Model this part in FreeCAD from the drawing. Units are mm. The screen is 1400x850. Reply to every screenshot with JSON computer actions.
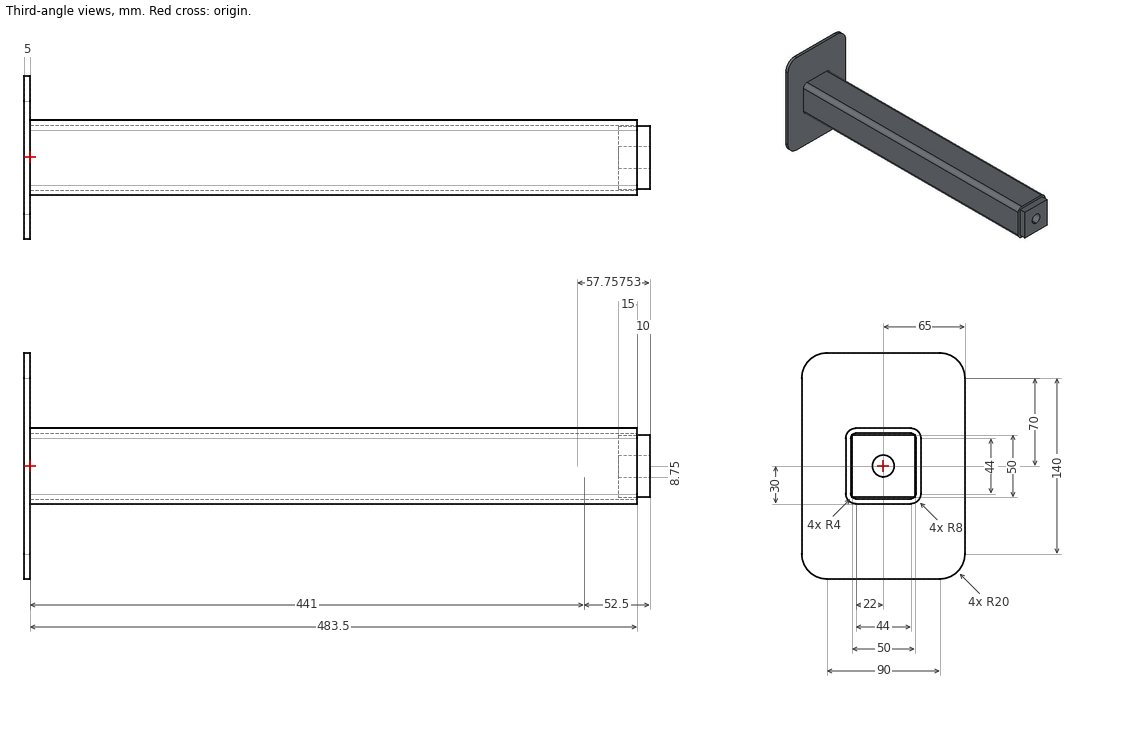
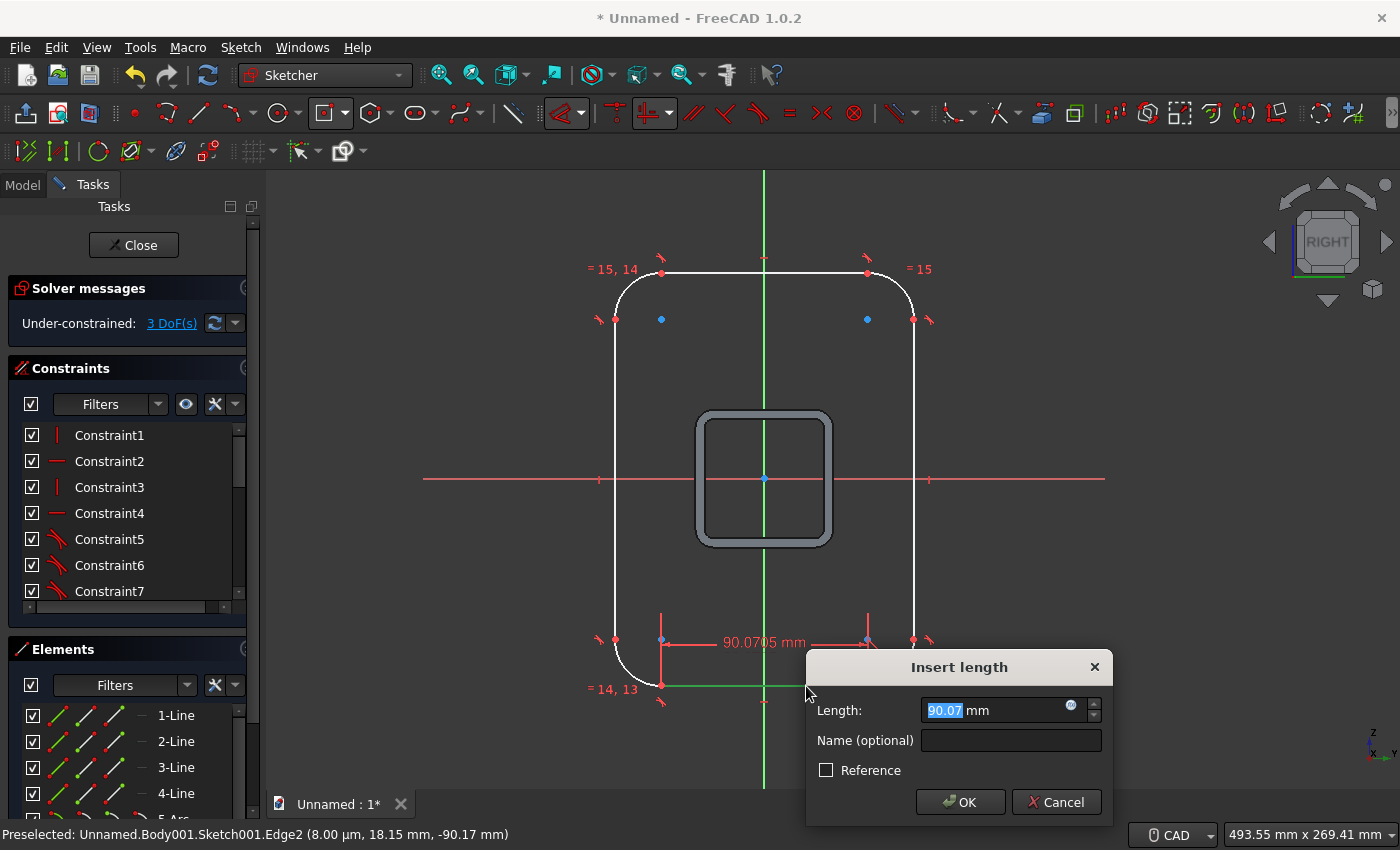
{"action": "type", "text": "90"}
{"action": "key", "text": "Return"}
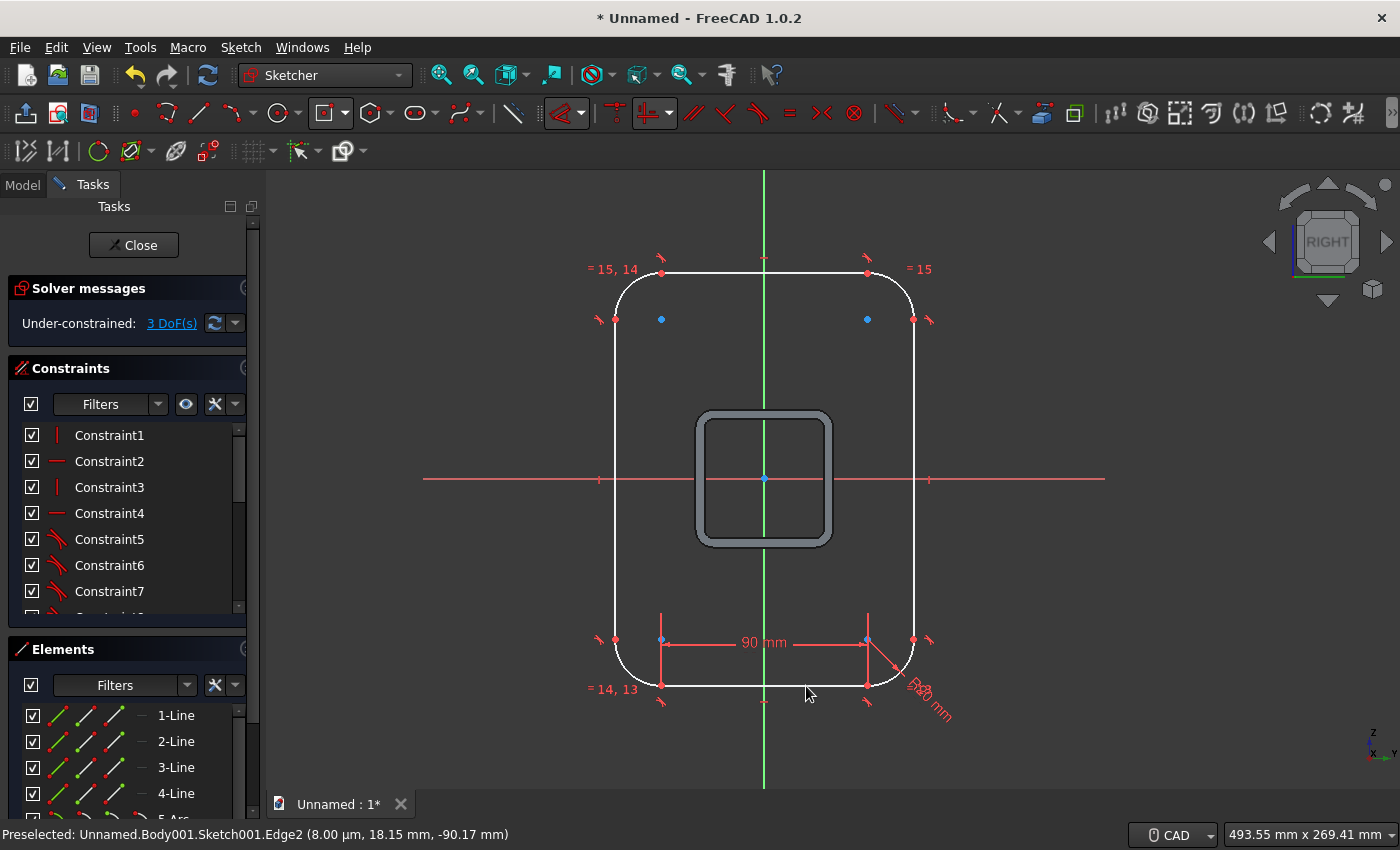
{"action": "left_click", "coordinate": [914, 415]}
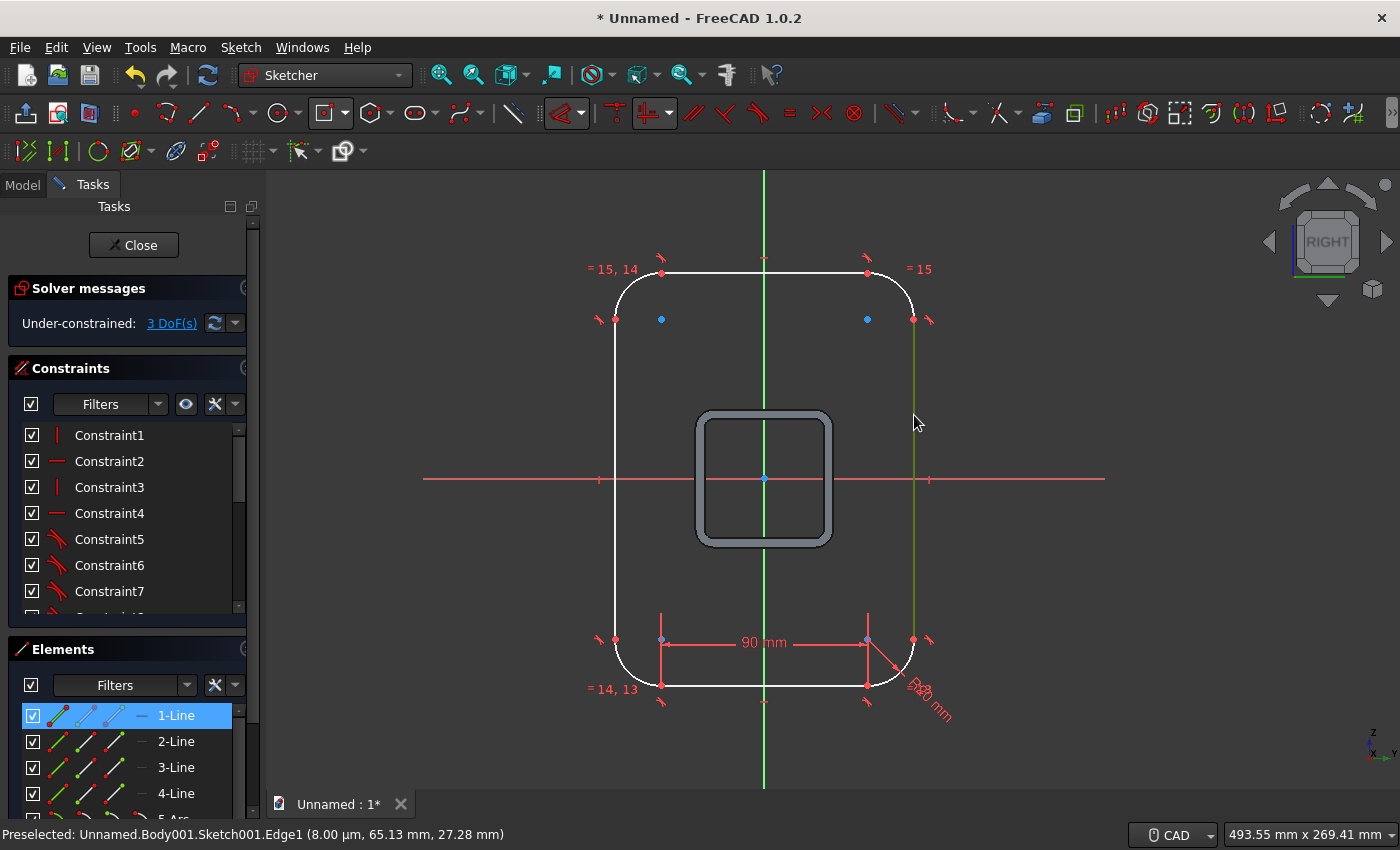
{"action": "key", "text": "i"}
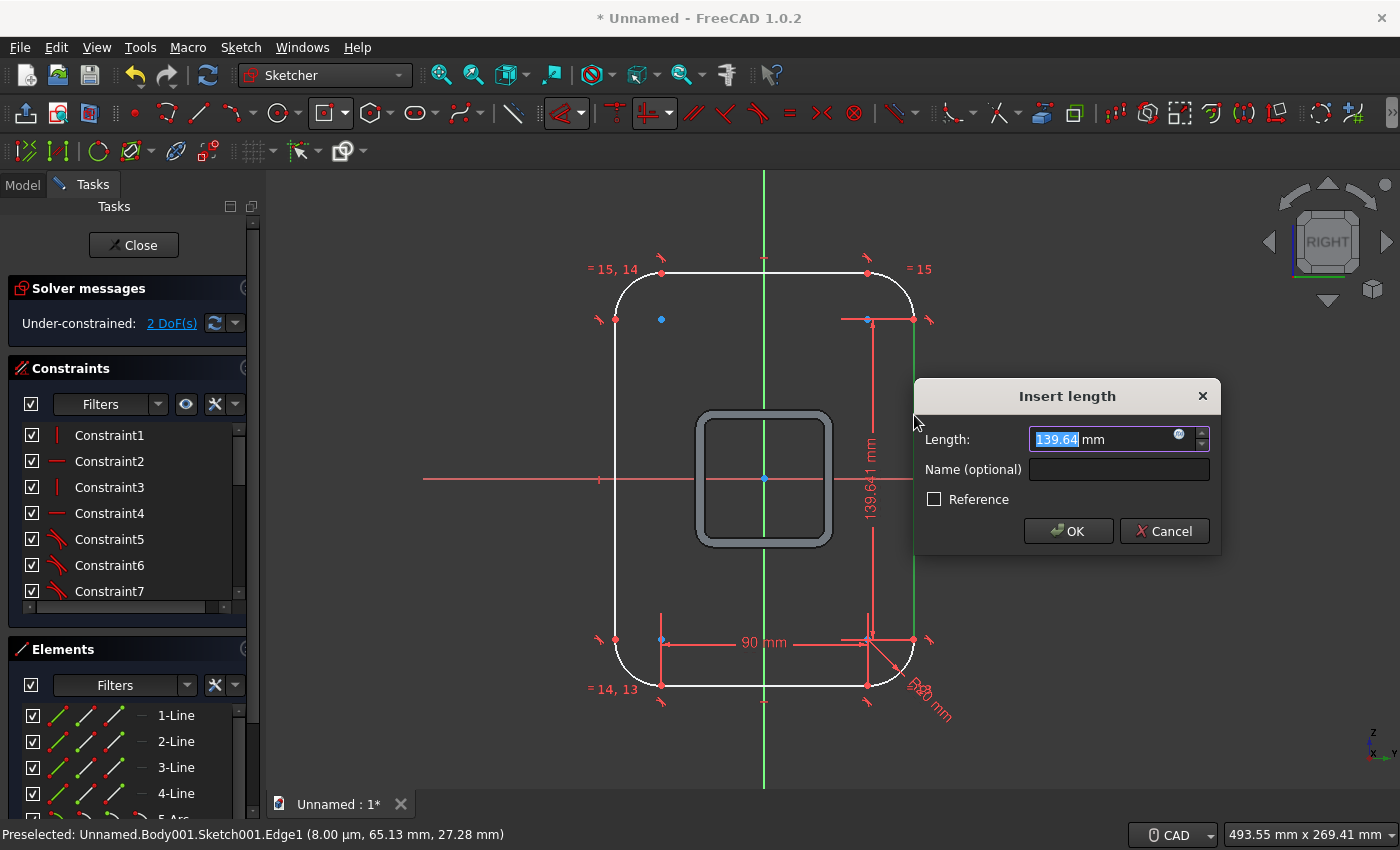
{"action": "type", "text": "140"}
{"action": "key", "text": "Return"}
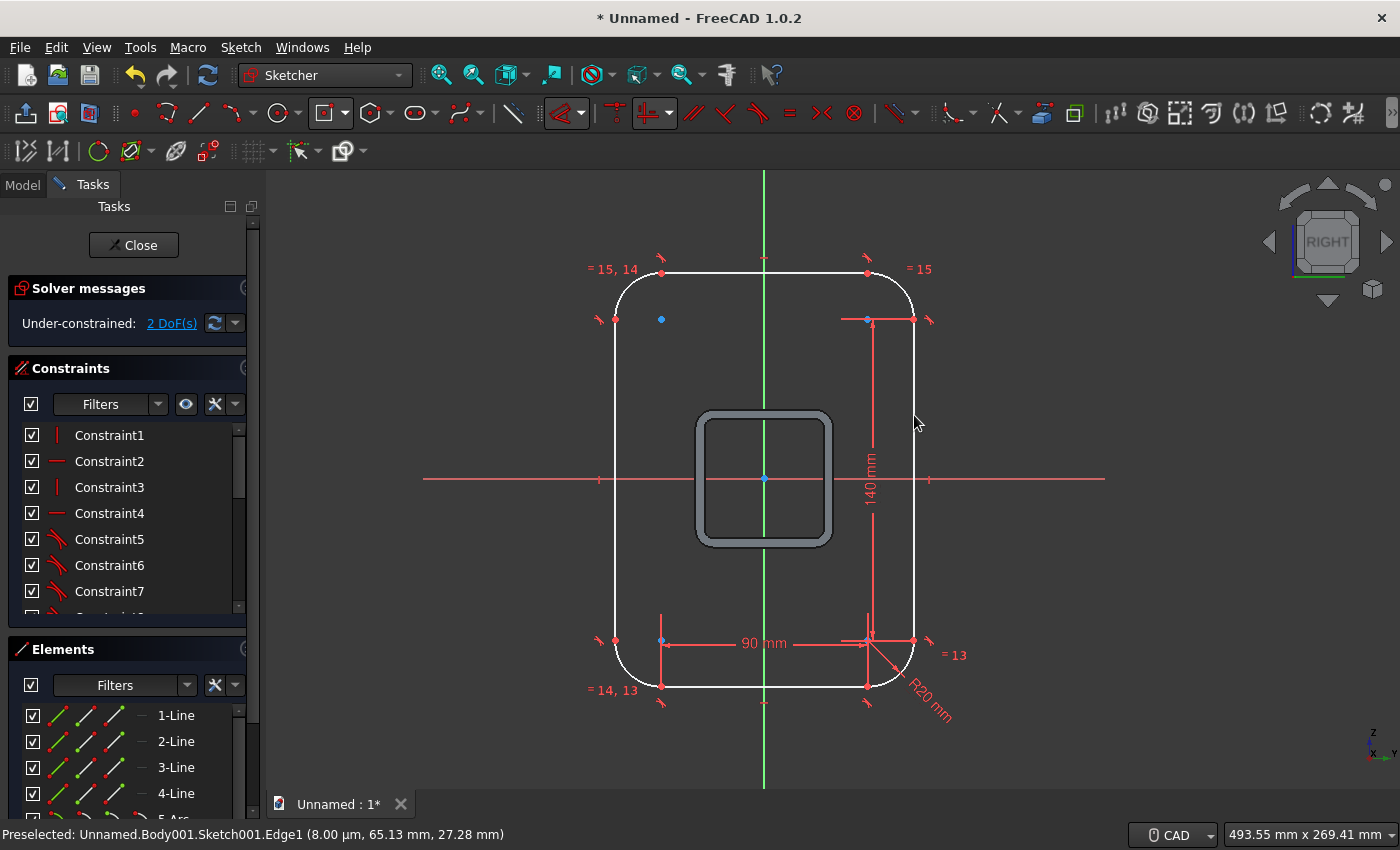
{"action": "left_click", "coordinate": [914, 319]}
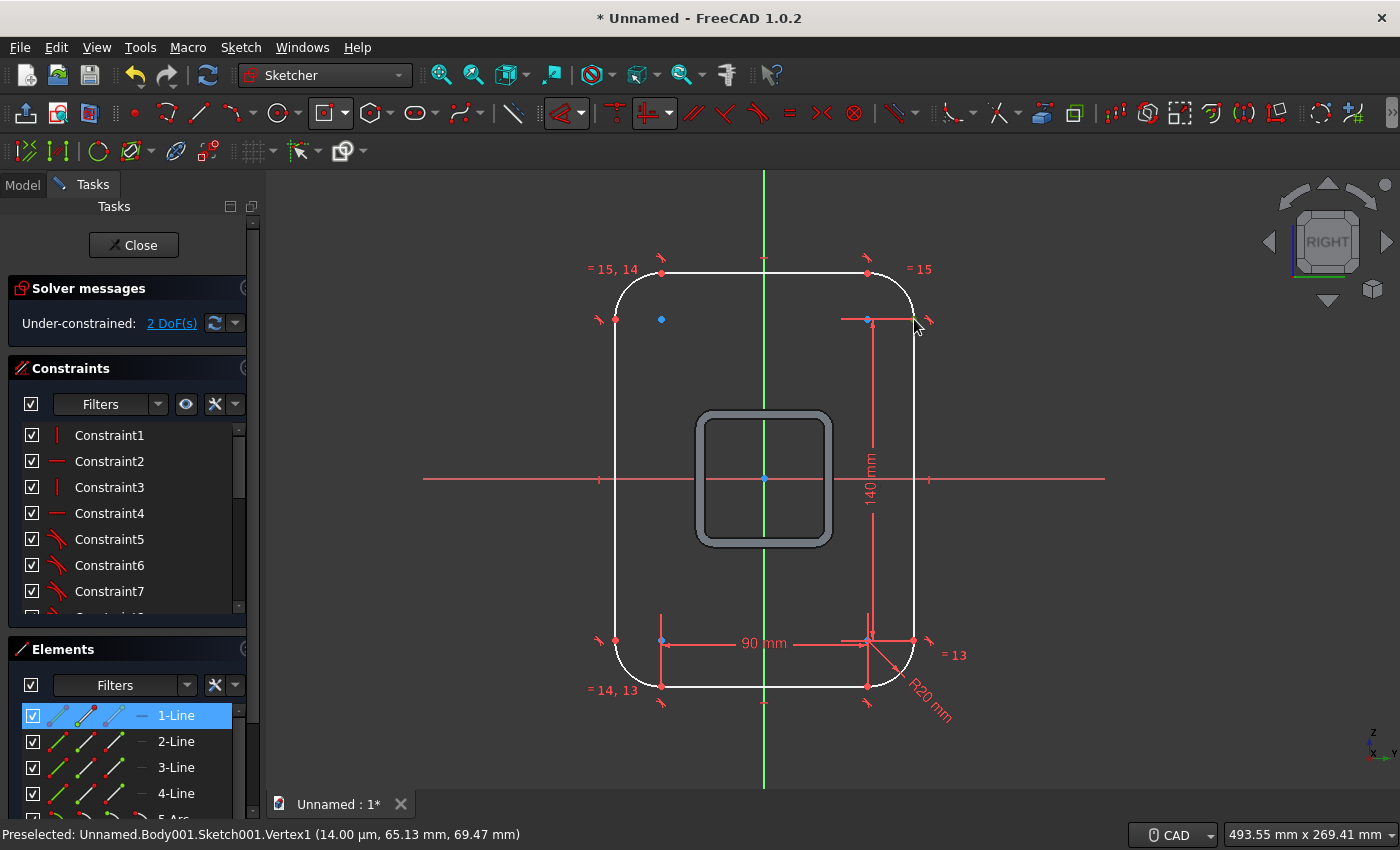
{"action": "left_click", "coordinate": [584, 114]}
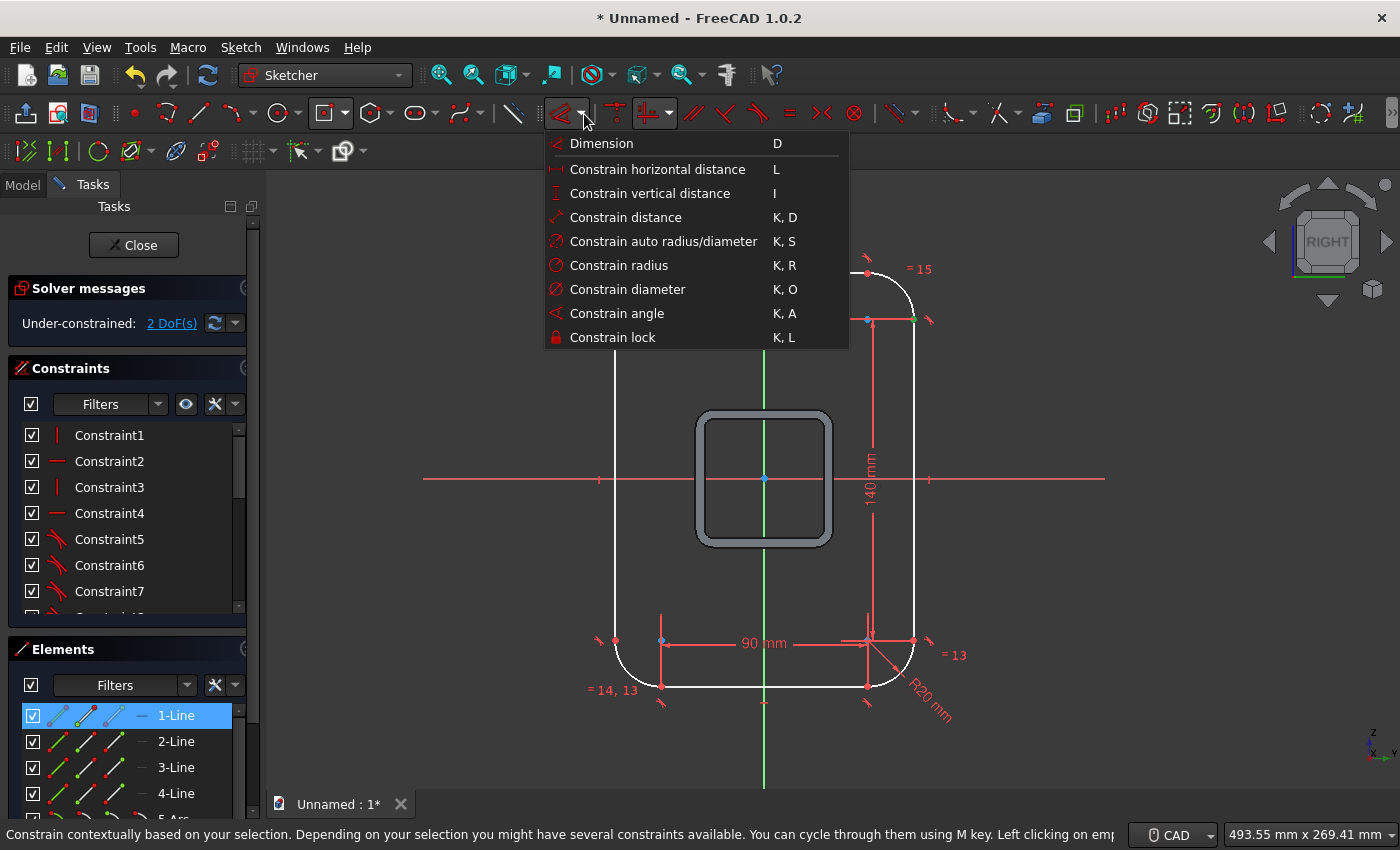
{"action": "left_click", "coordinate": [697, 169]}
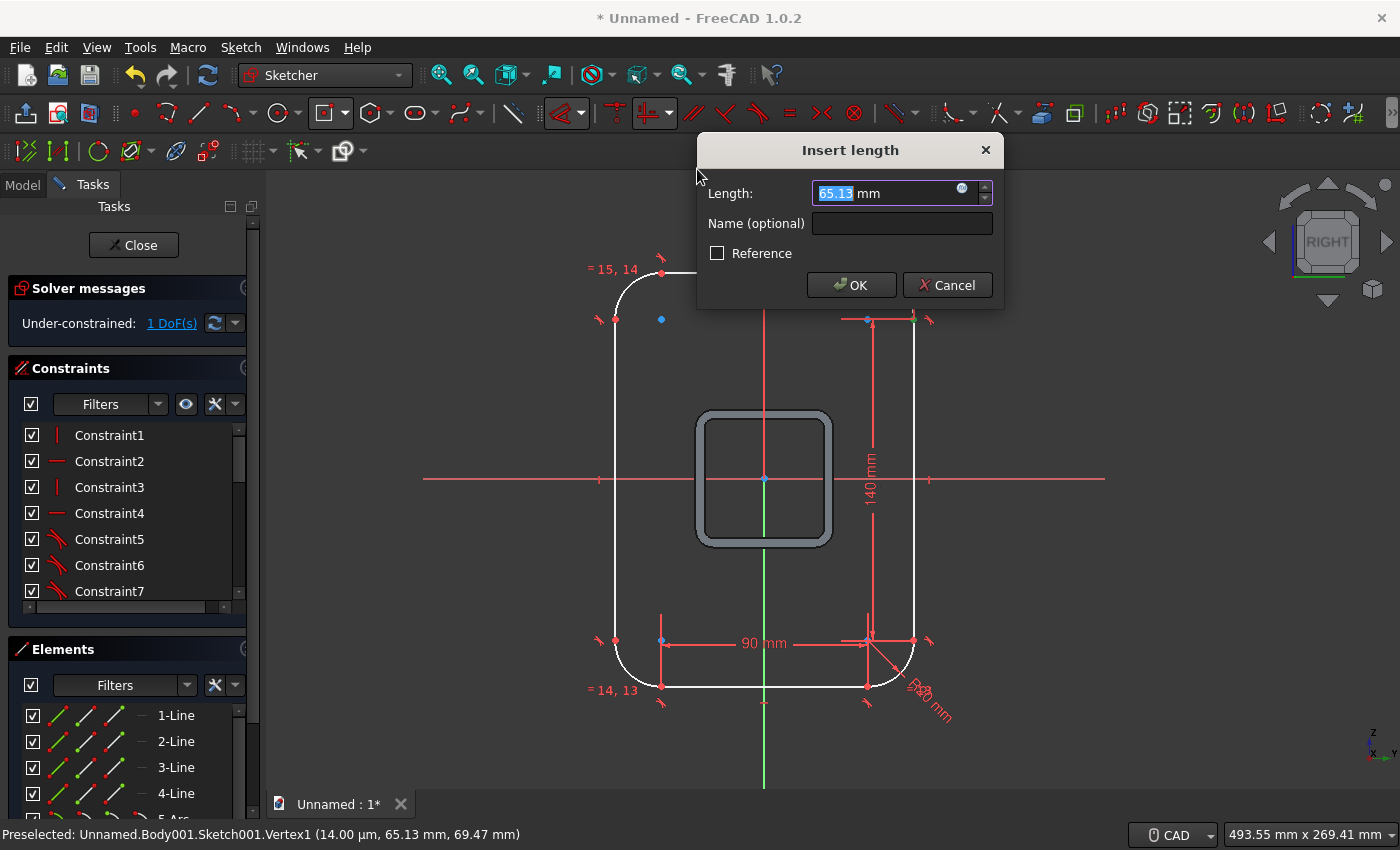
{"action": "type", "text": "65"}
{"action": "key", "text": "Return"}